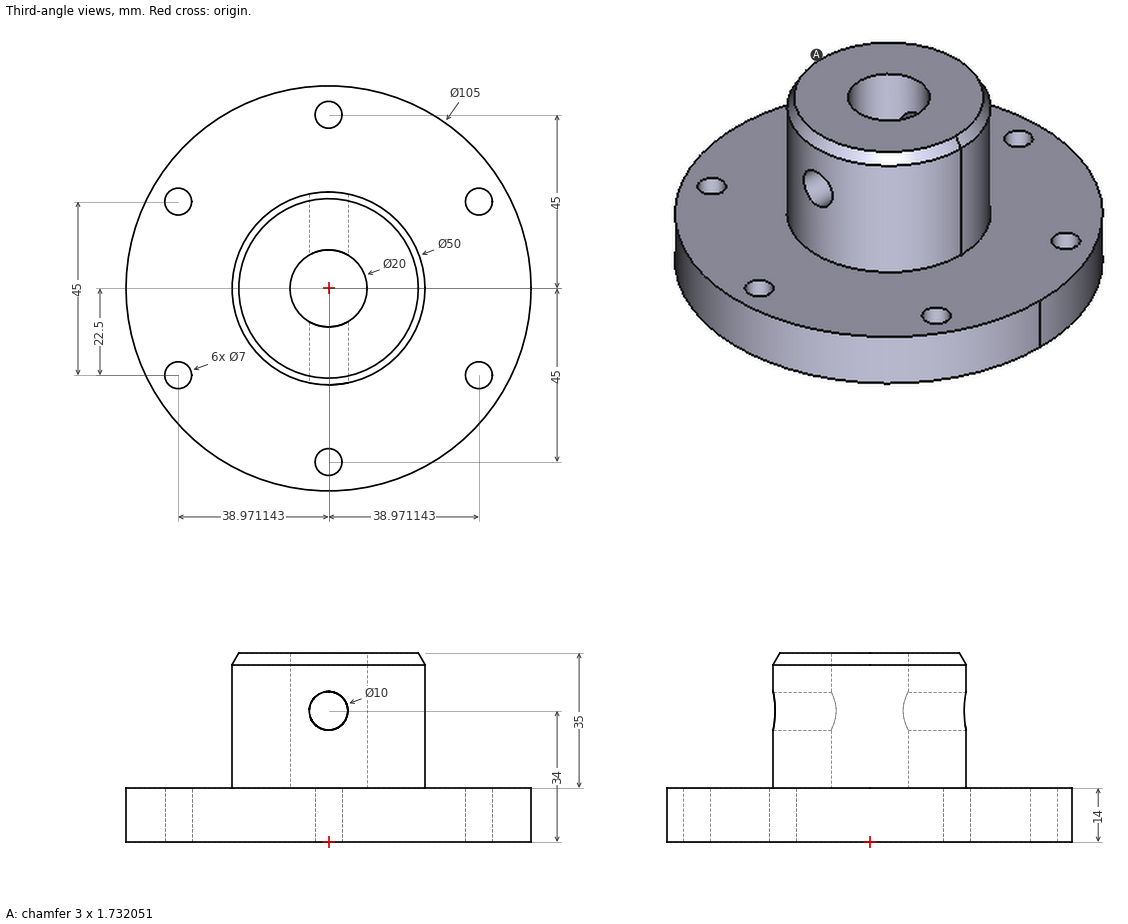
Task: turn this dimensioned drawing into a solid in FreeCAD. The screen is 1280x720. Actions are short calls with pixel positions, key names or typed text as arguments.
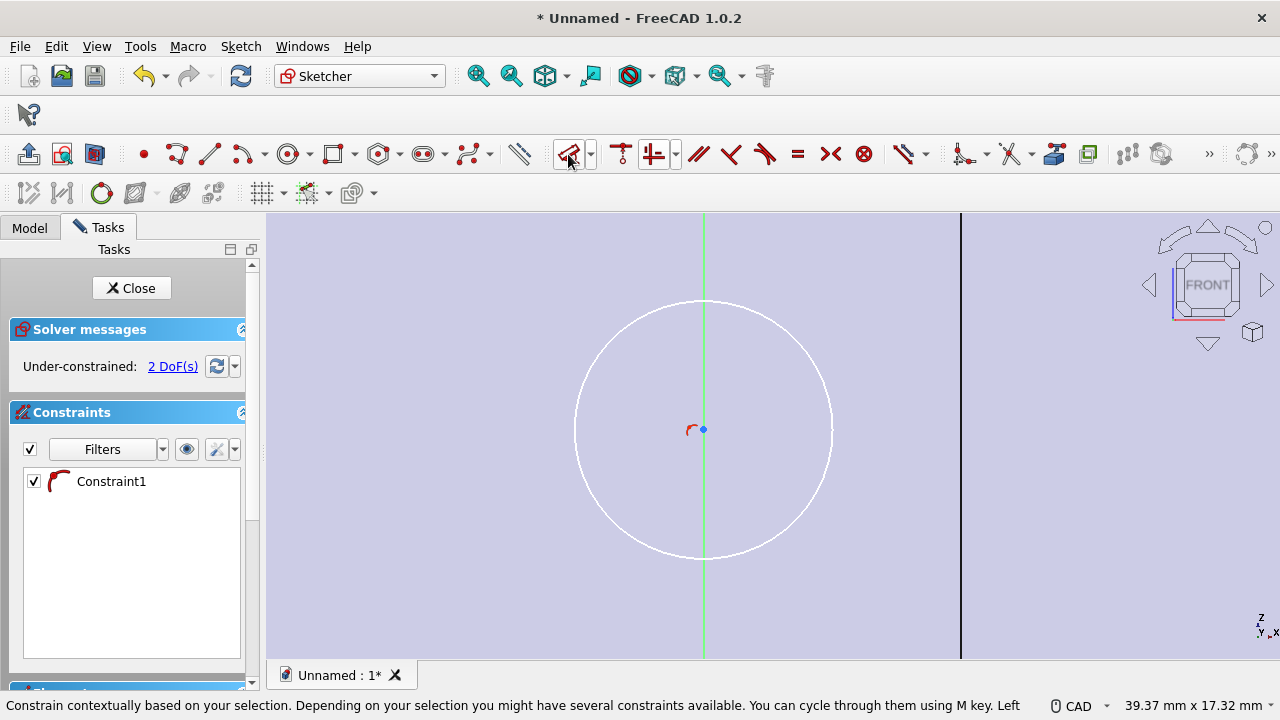
click(795, 339)
click(818, 316)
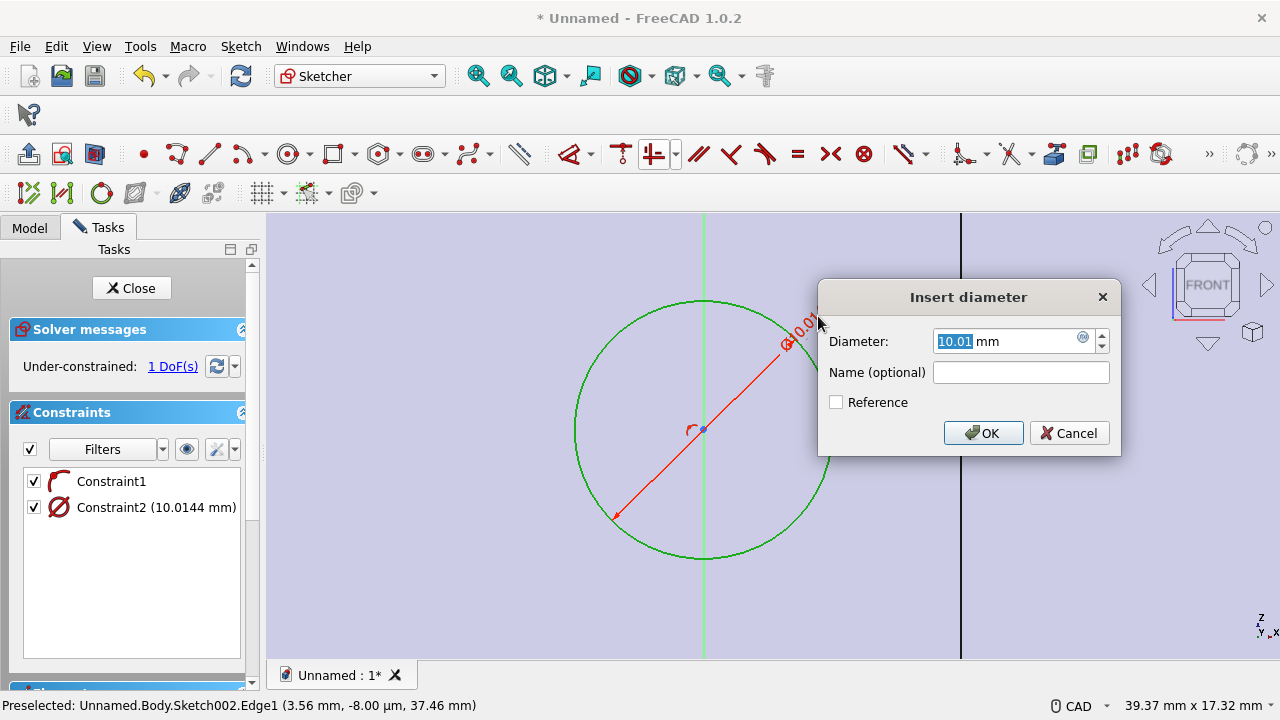
text(10)
key(Return)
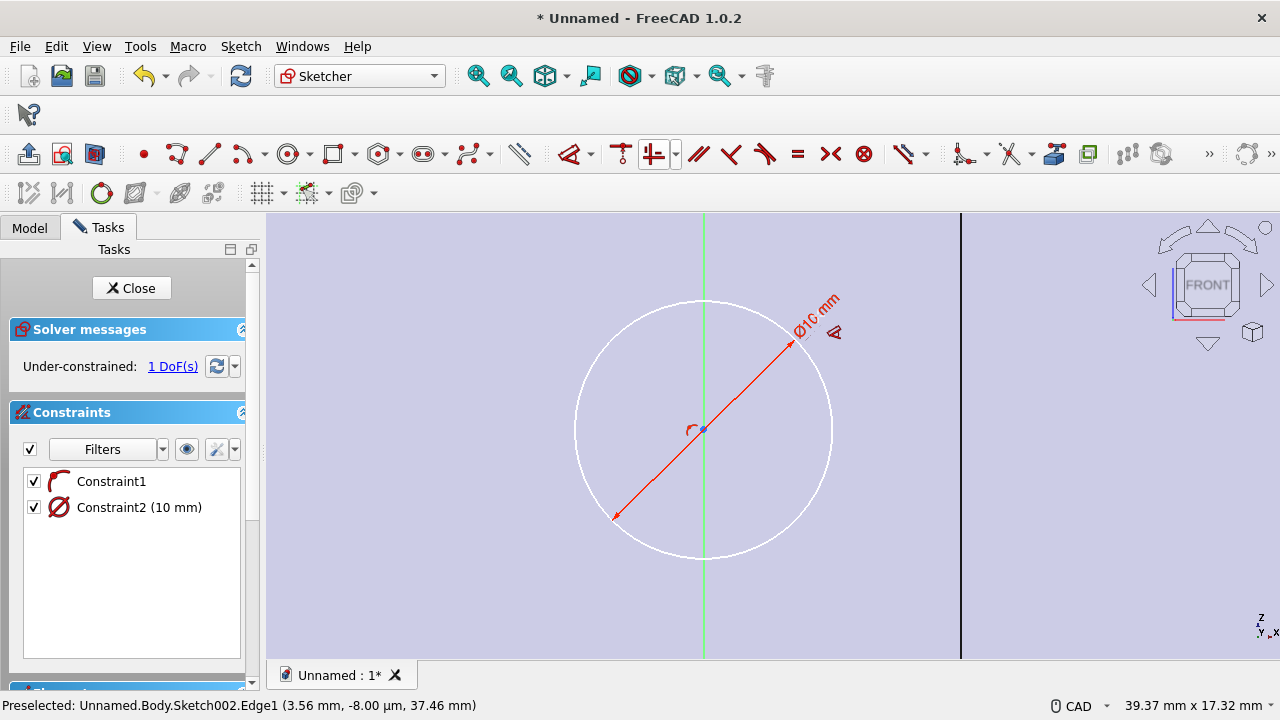
click(704, 430)
click(738, 531)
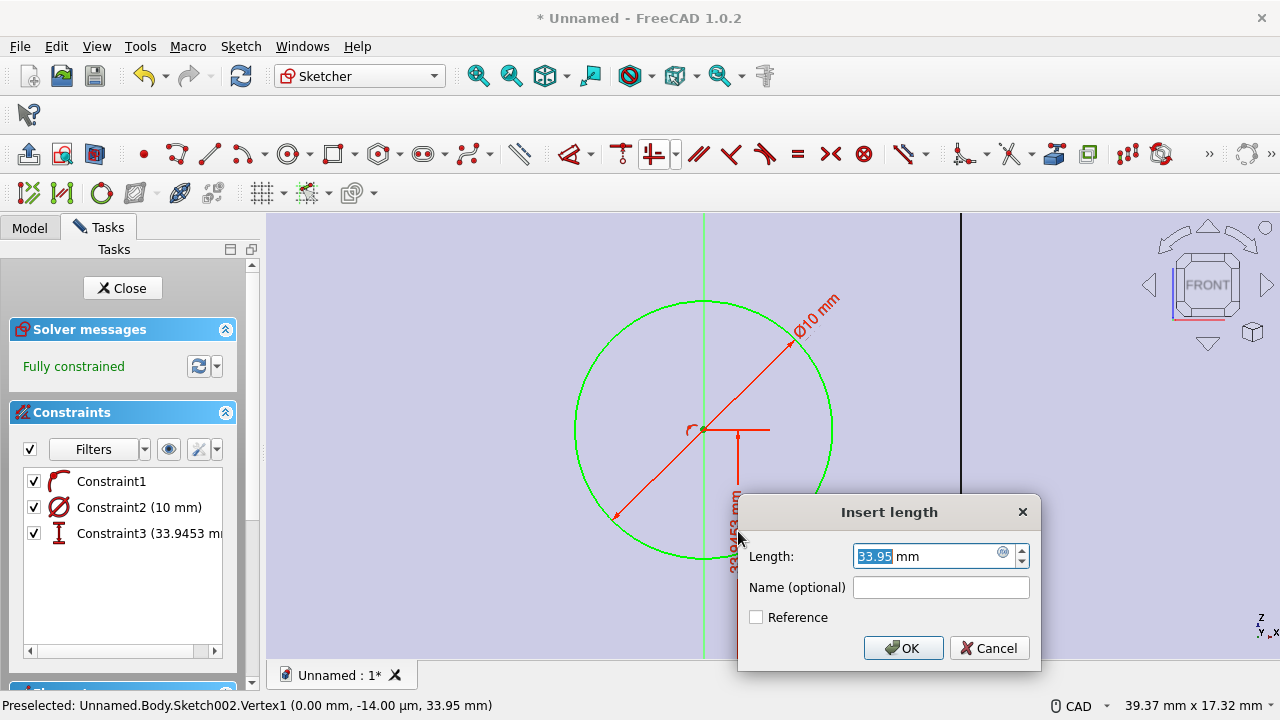
text(34)
key(Return)
key(Escape)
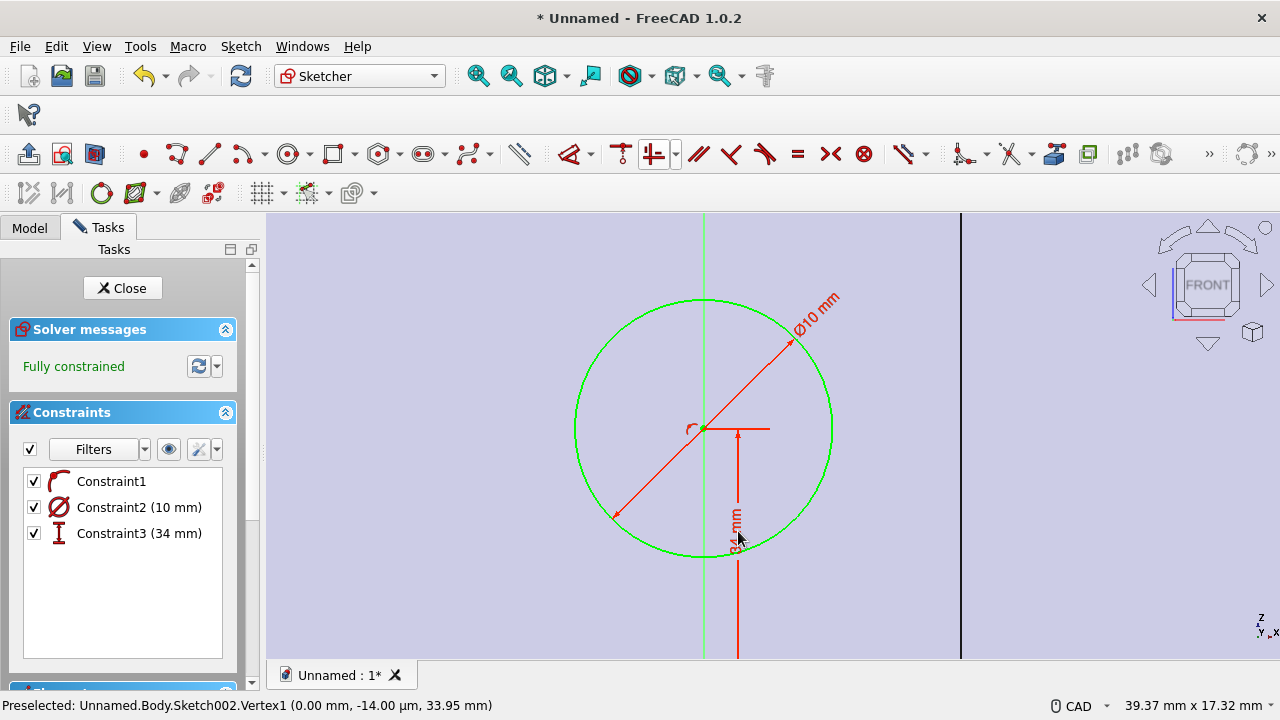
click(123, 288)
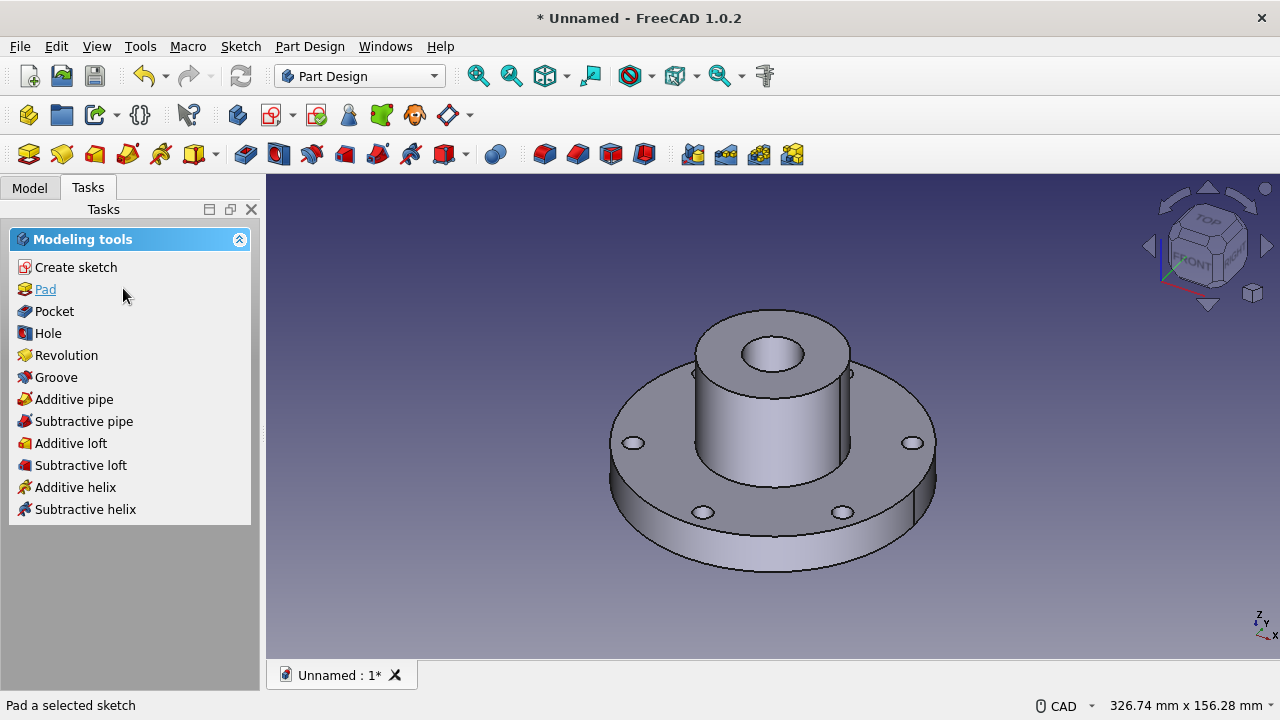
click(246, 154)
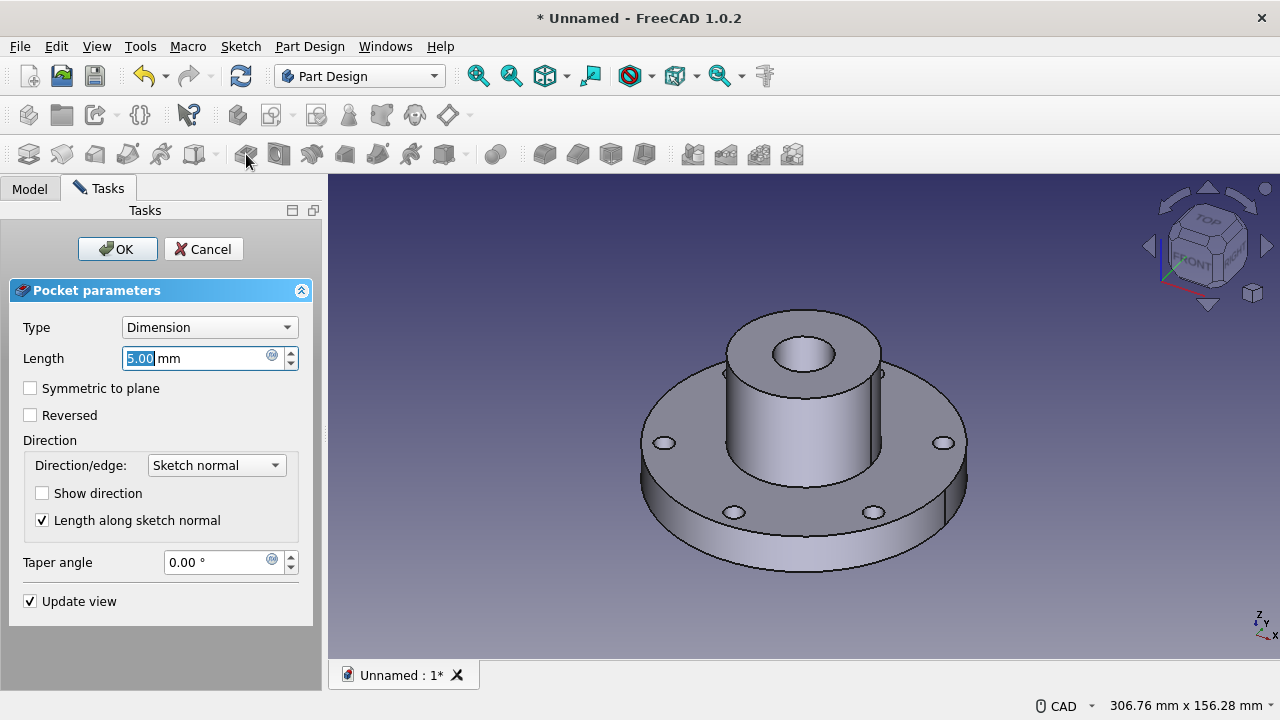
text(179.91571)
key(Tab)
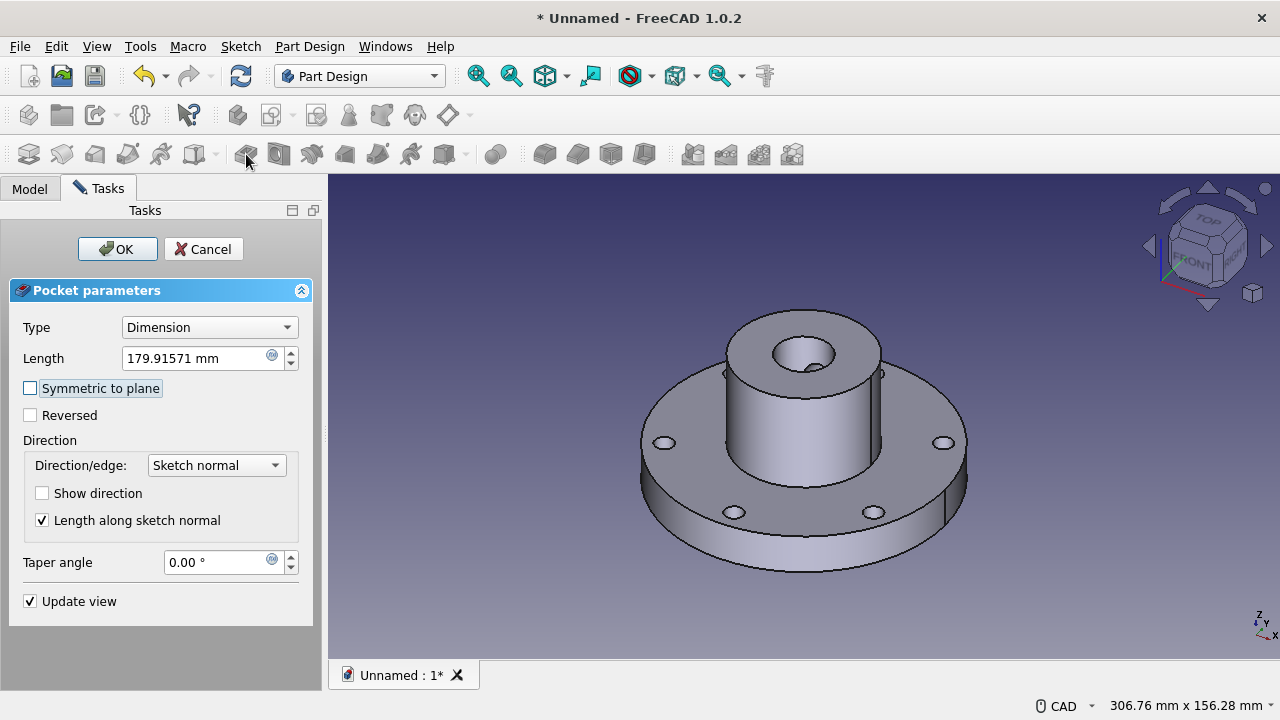
click(31, 388)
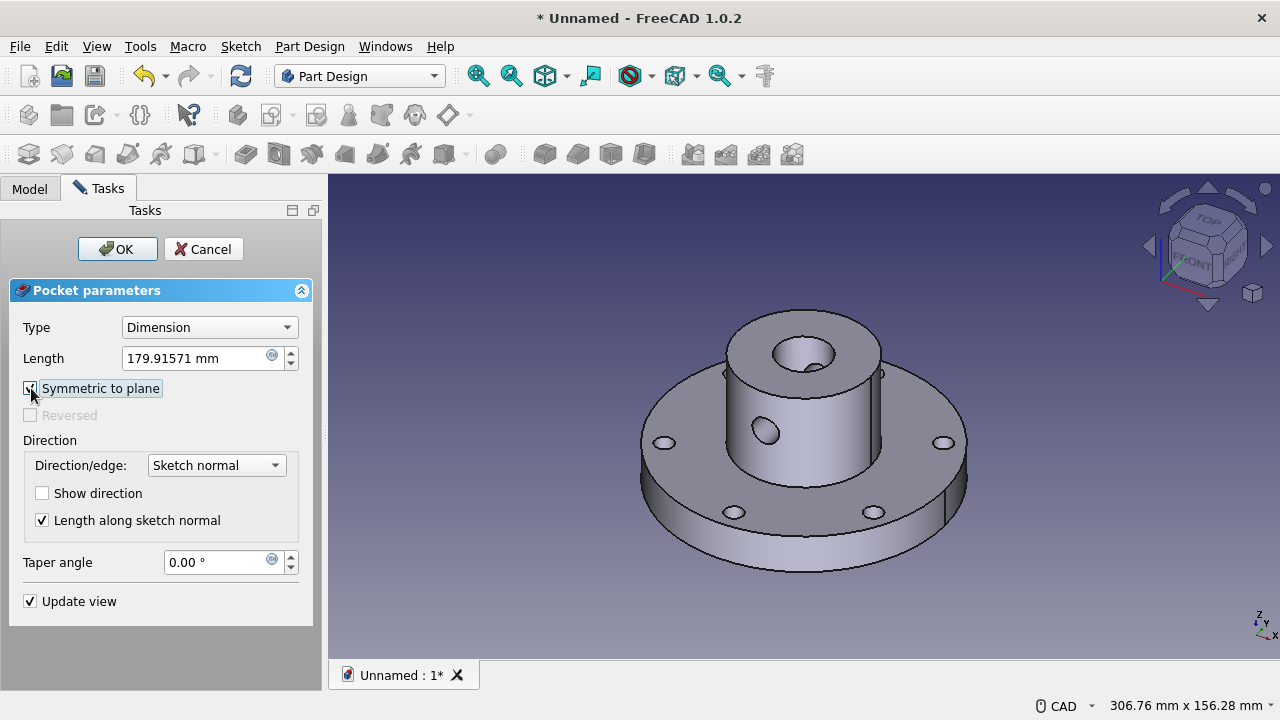
click(118, 249)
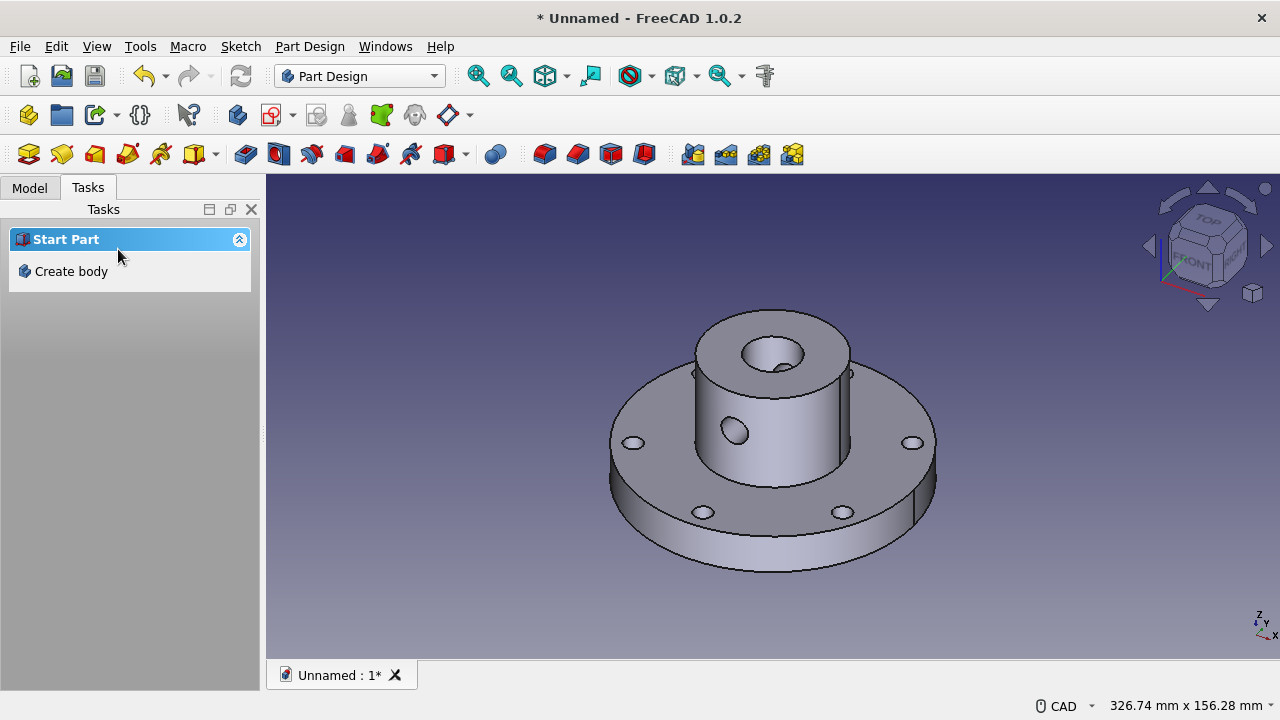
click(696, 358)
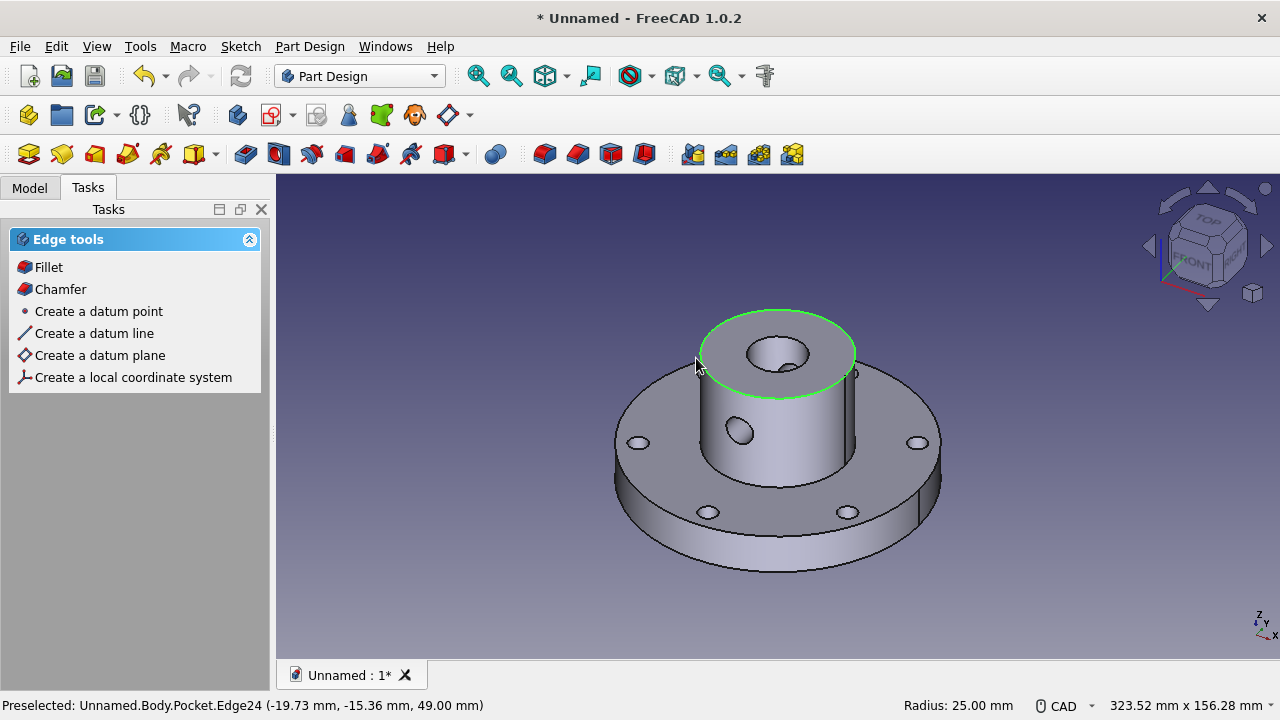
click(578, 154)